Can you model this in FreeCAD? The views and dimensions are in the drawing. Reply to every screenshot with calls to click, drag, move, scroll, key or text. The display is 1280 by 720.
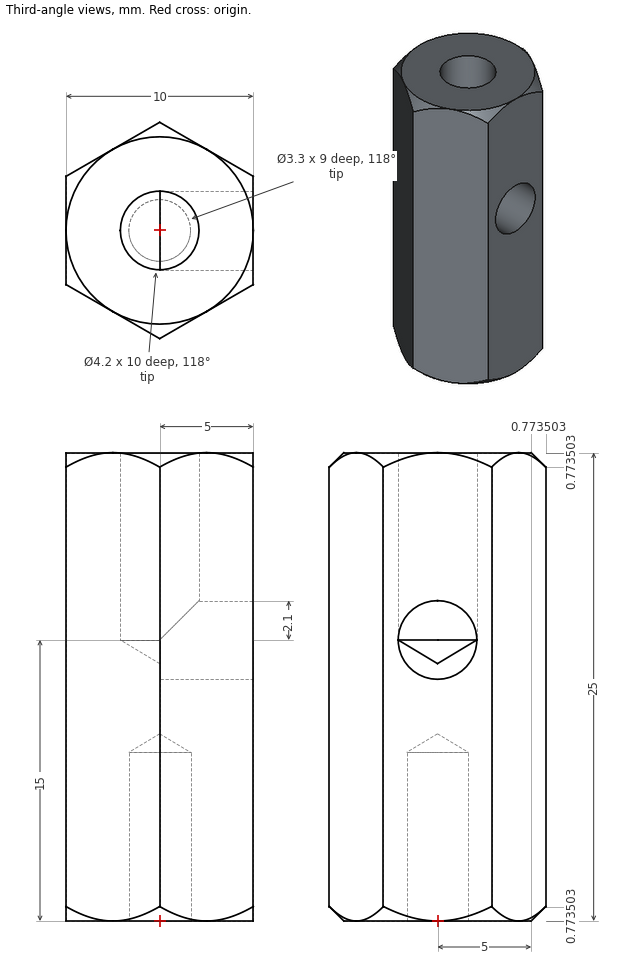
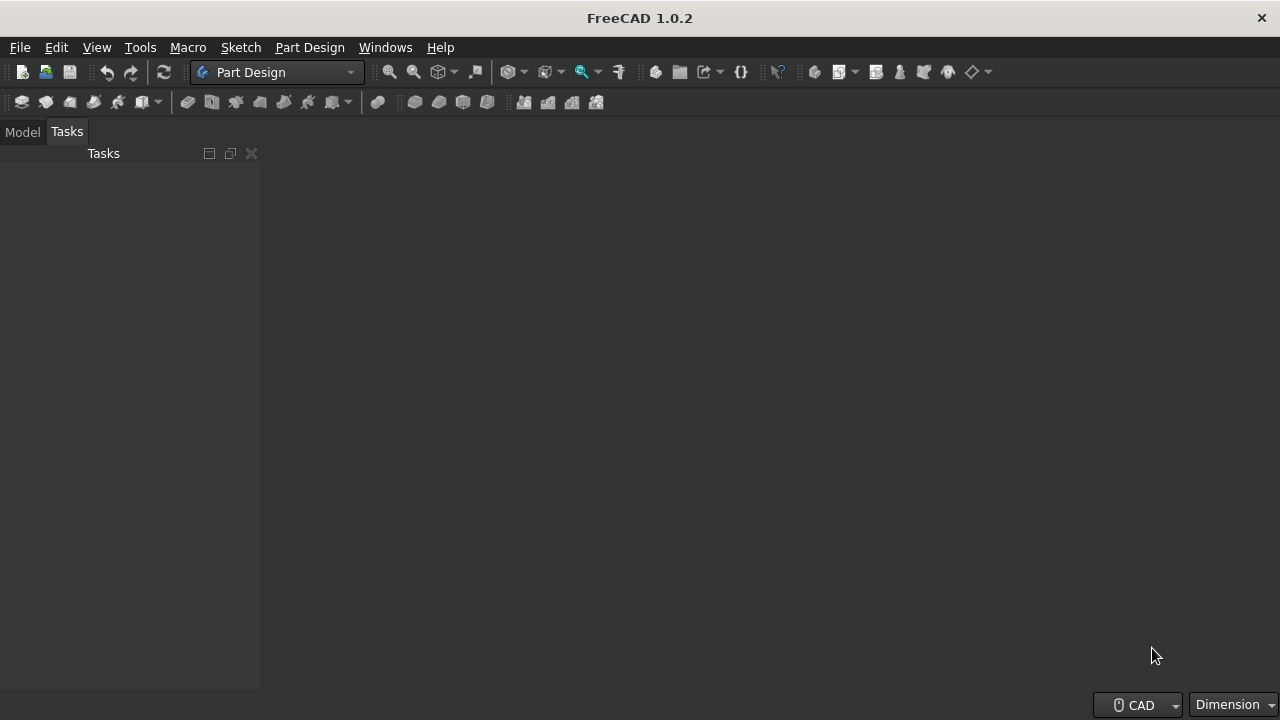
key(ctrl+n)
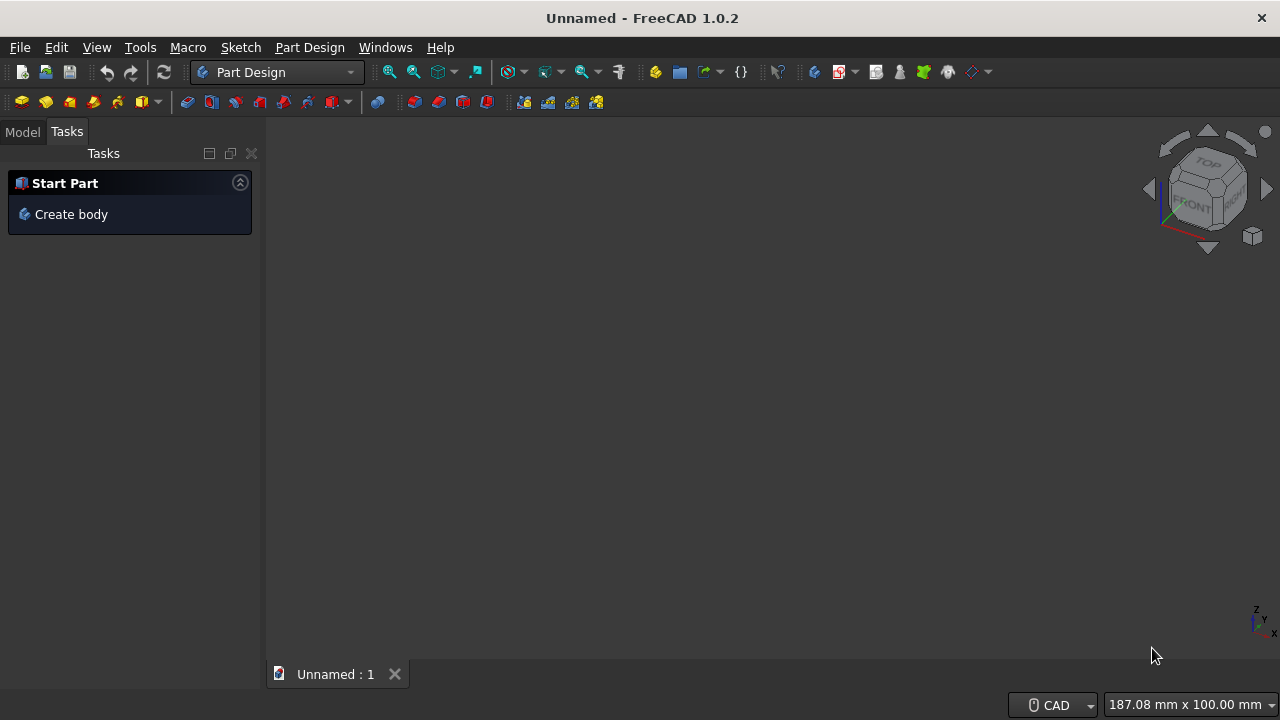
click(840, 72)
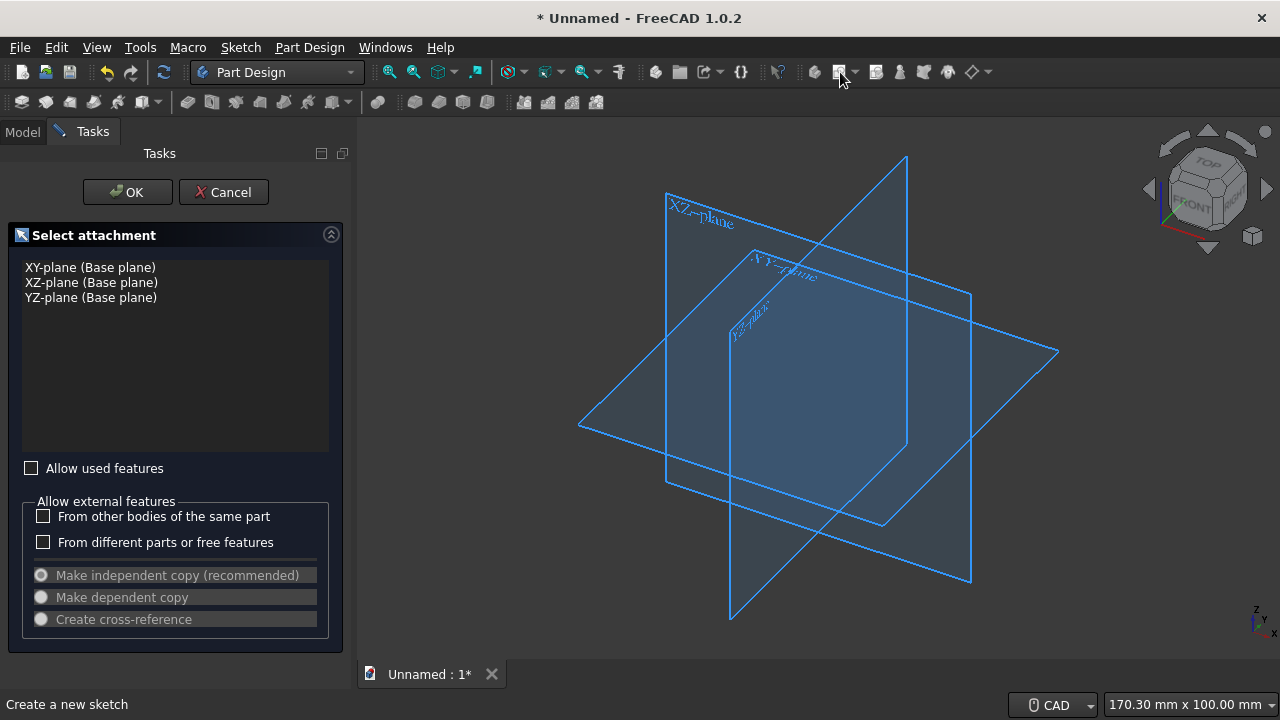
click(82, 268)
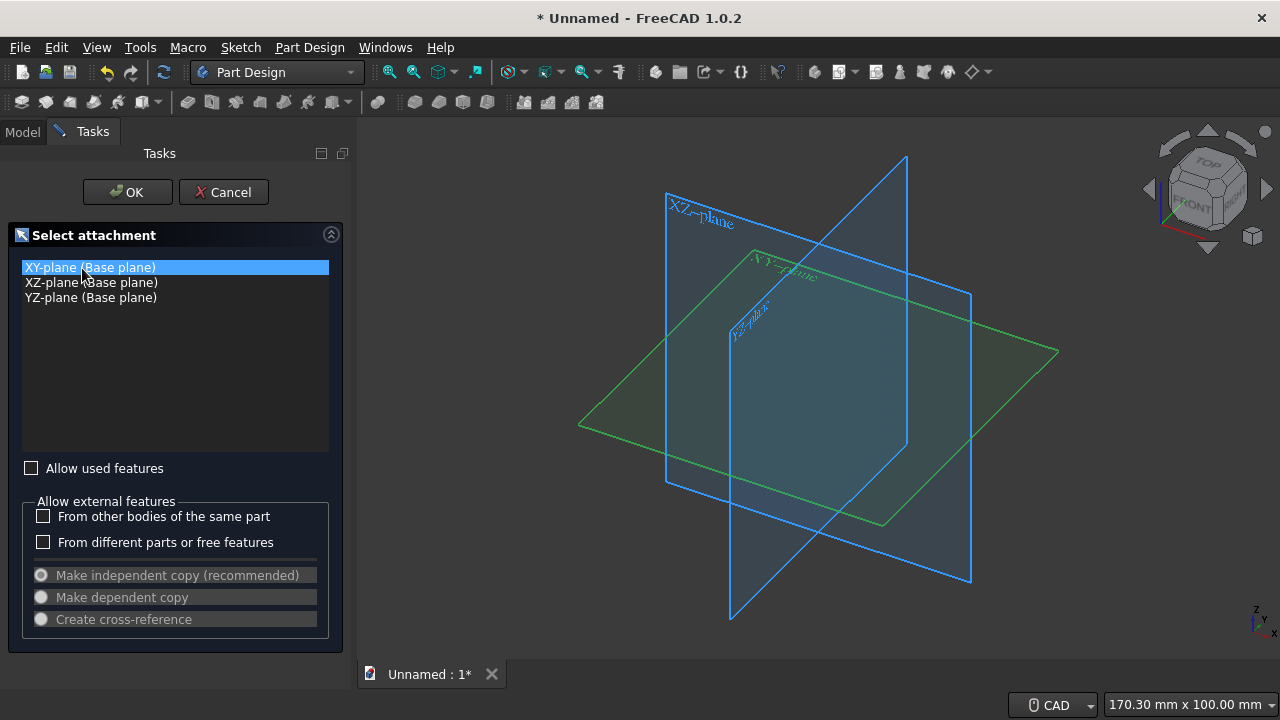
click(128, 192)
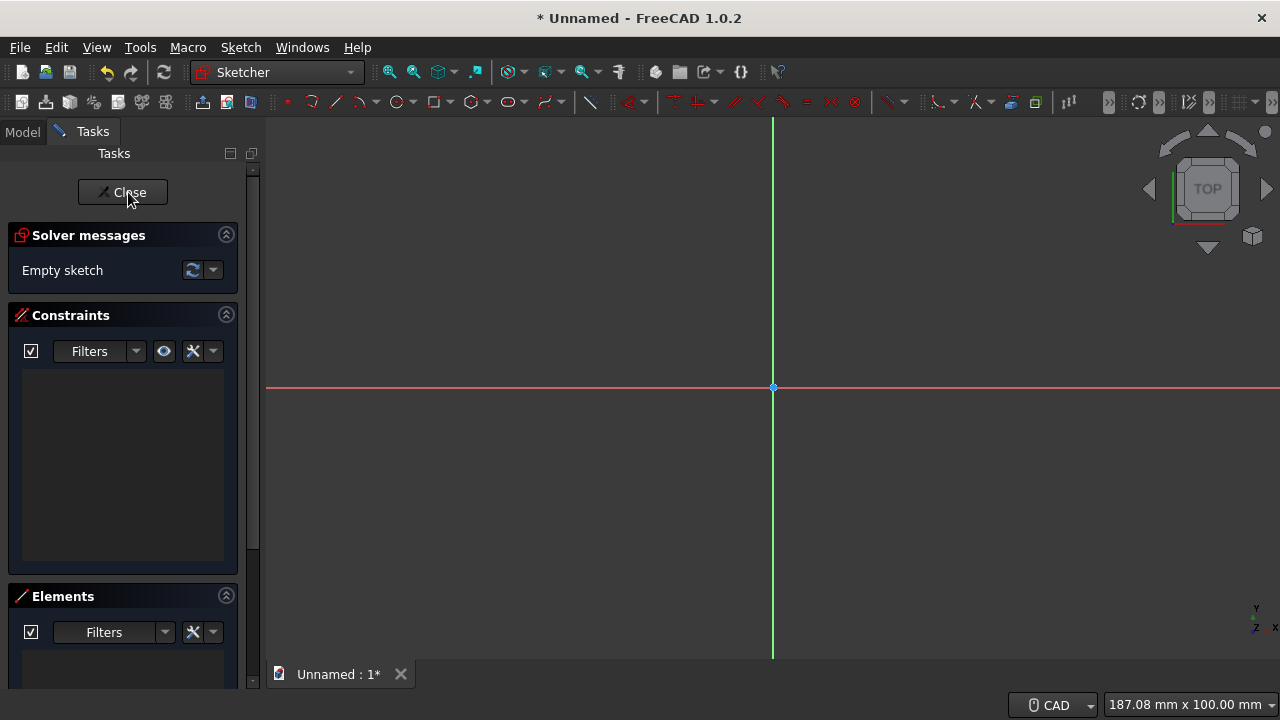
scroll(787, 388, up, 9)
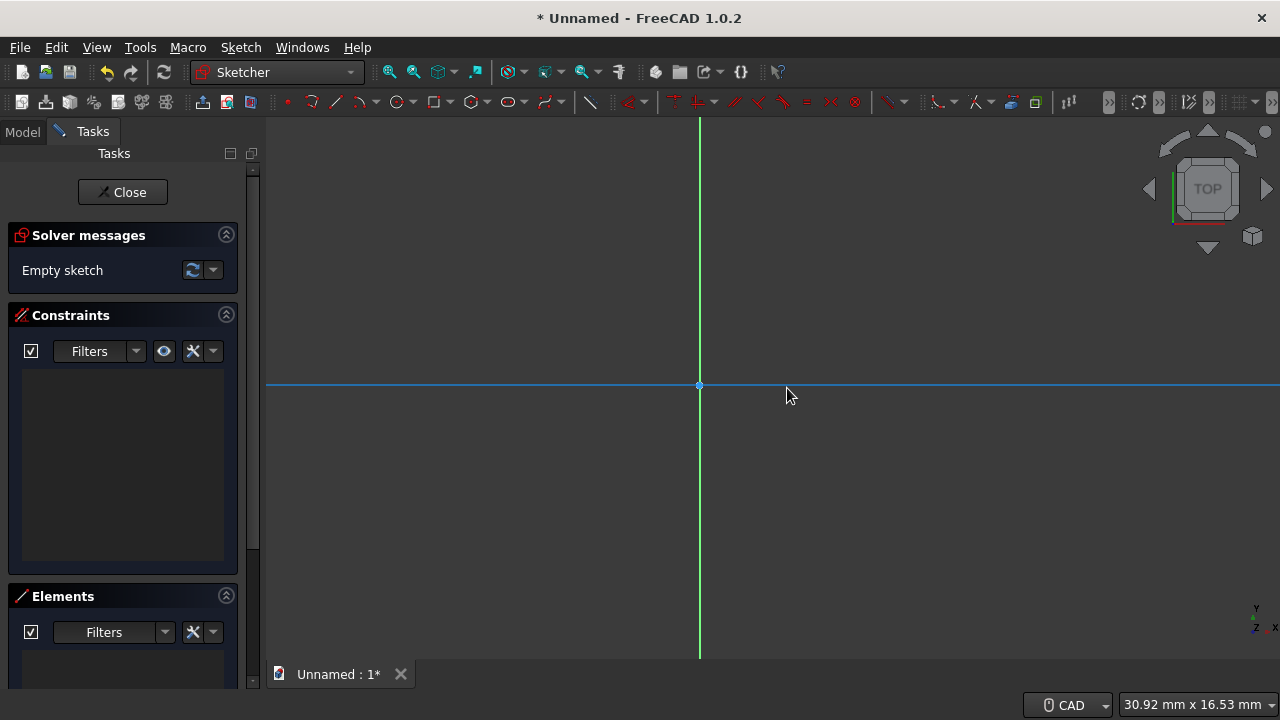
click(472, 102)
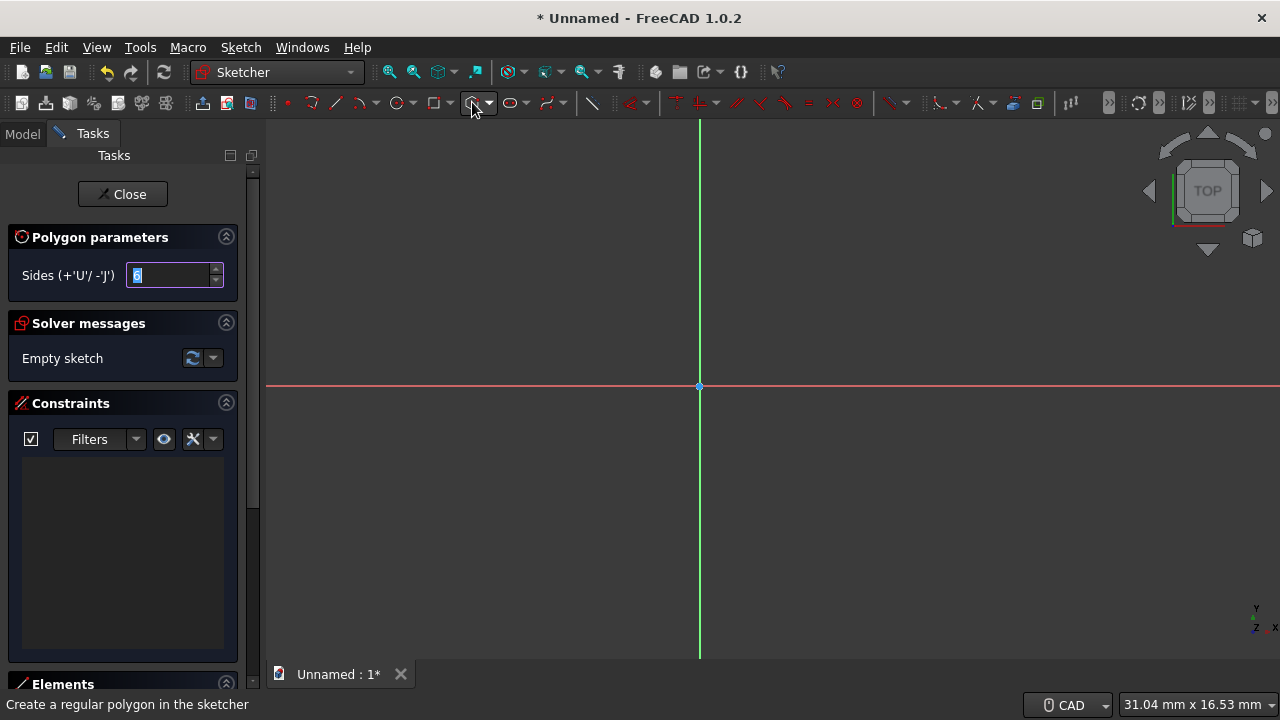
click(700, 386)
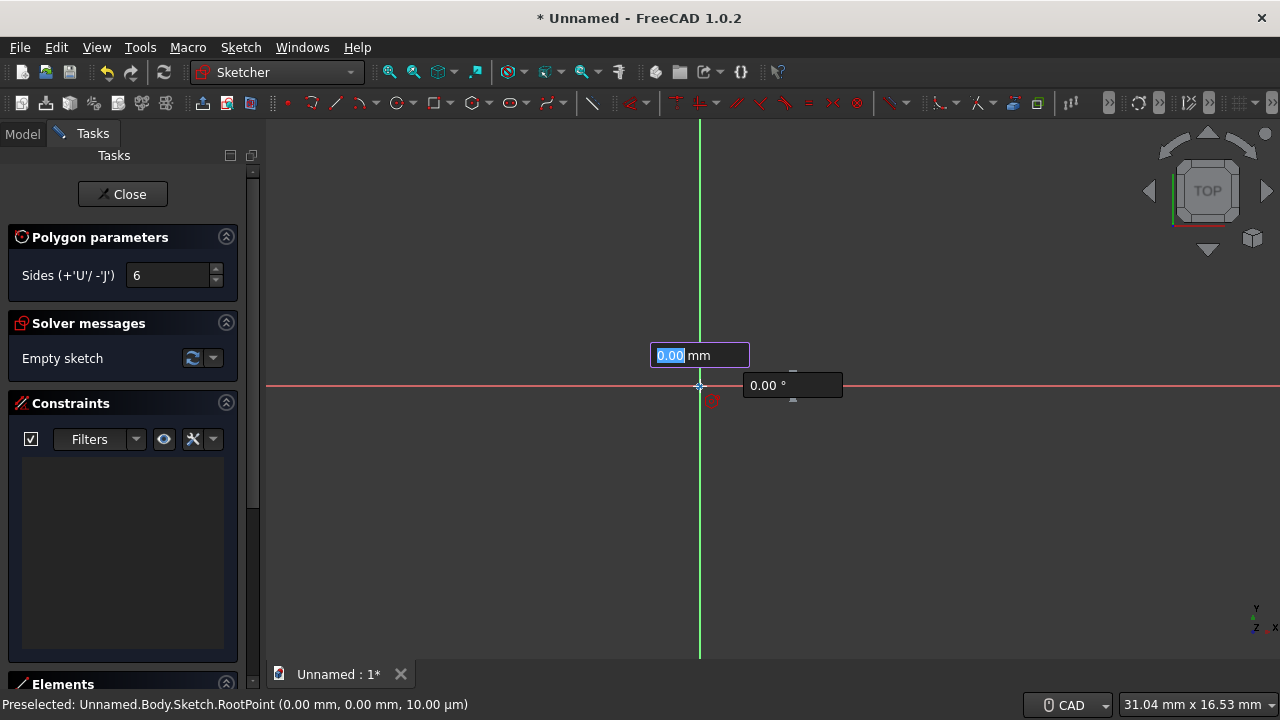
click(700, 198)
right_click(700, 198)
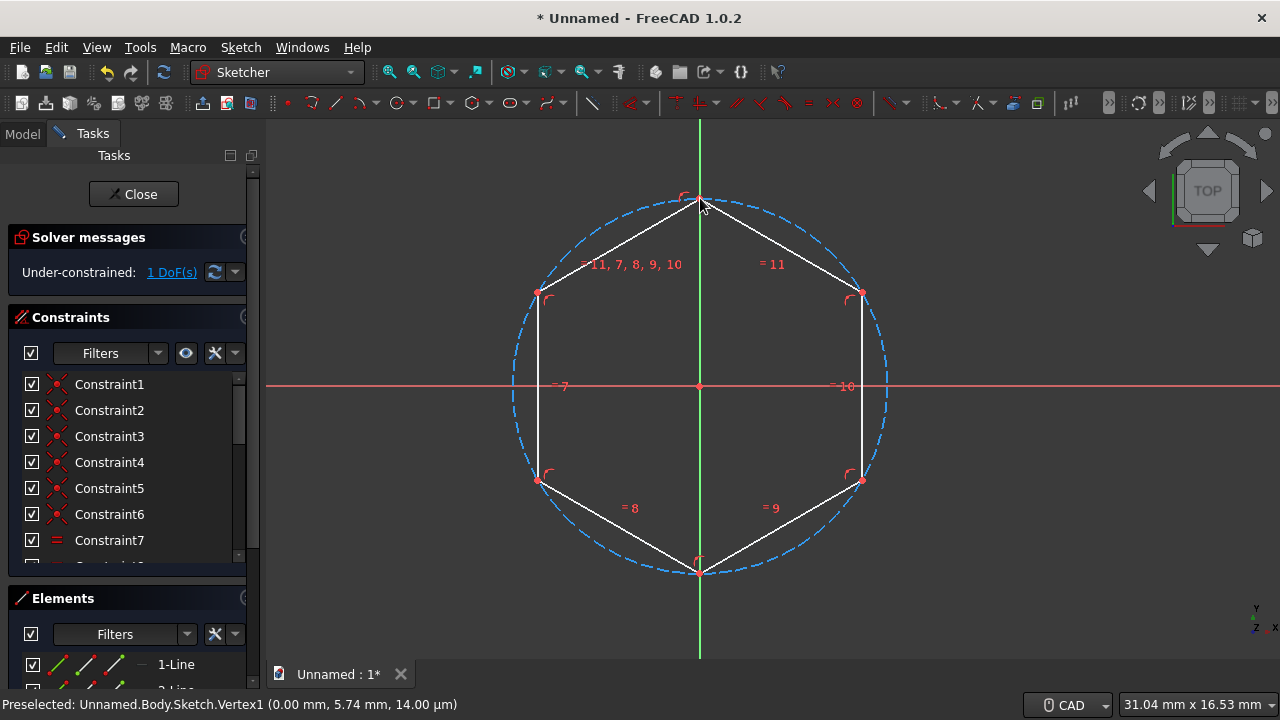
click(630, 104)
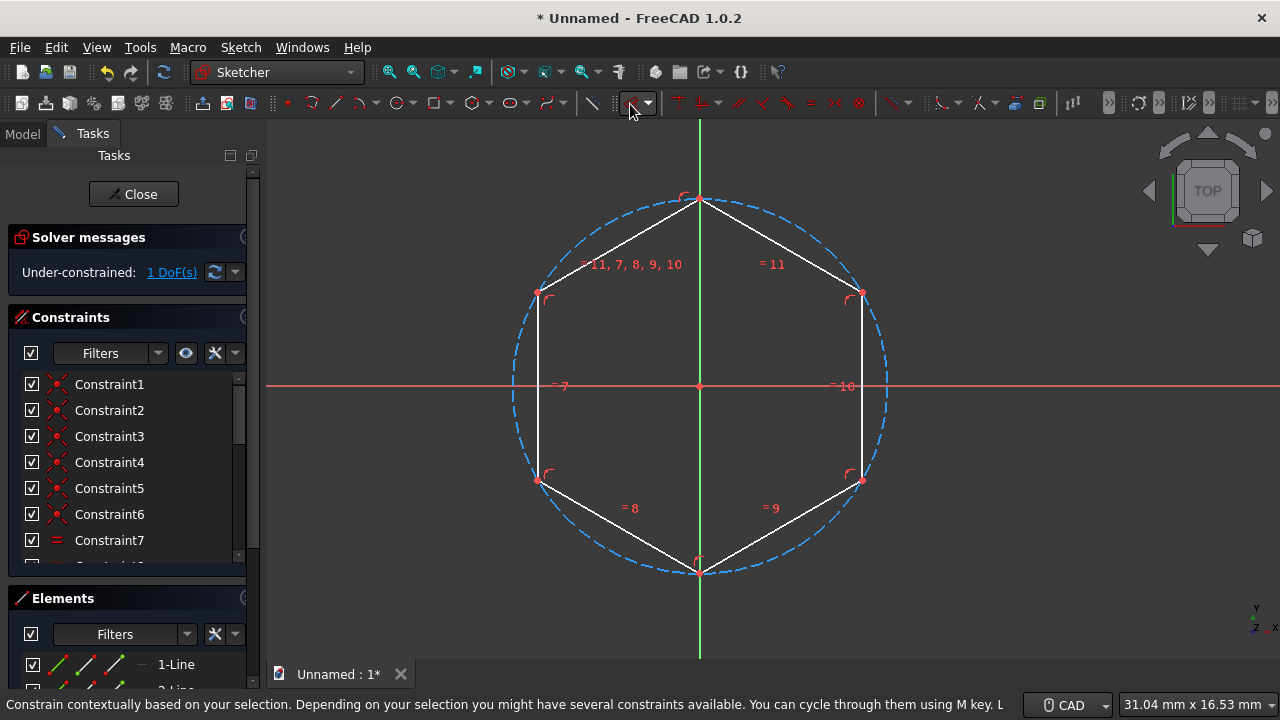
click(538, 293)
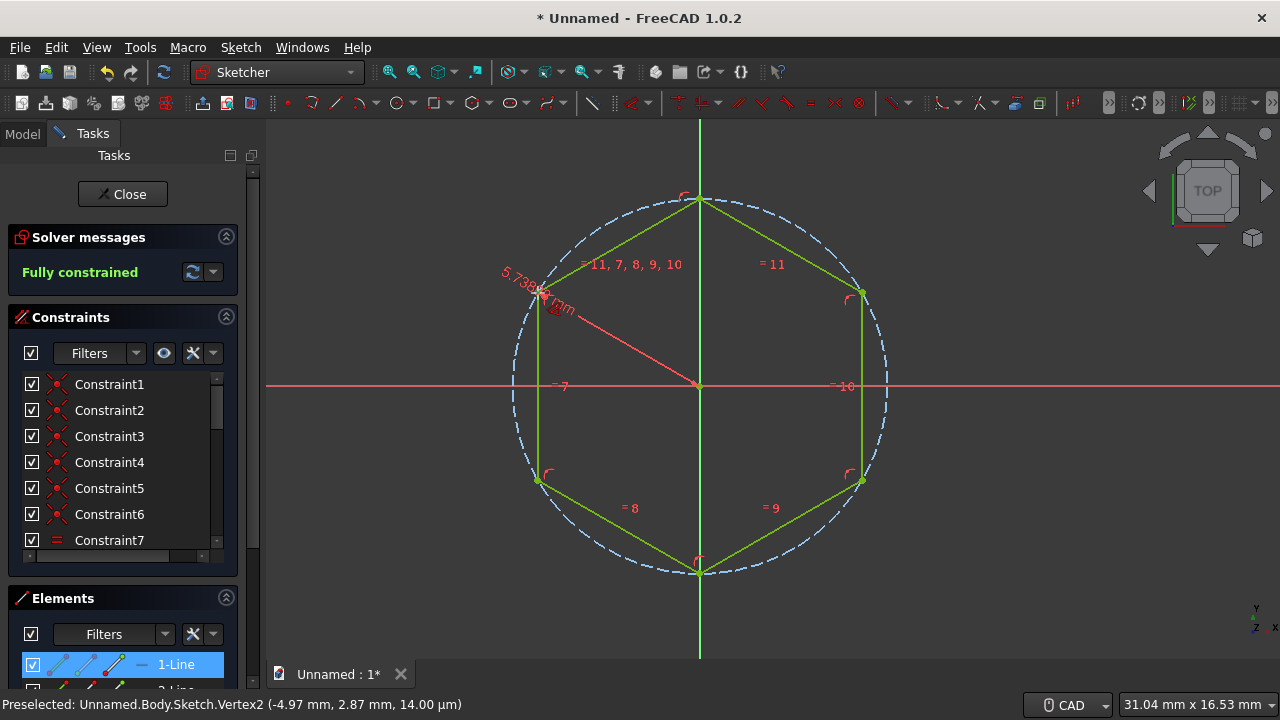
click(862, 480)
click(625, 514)